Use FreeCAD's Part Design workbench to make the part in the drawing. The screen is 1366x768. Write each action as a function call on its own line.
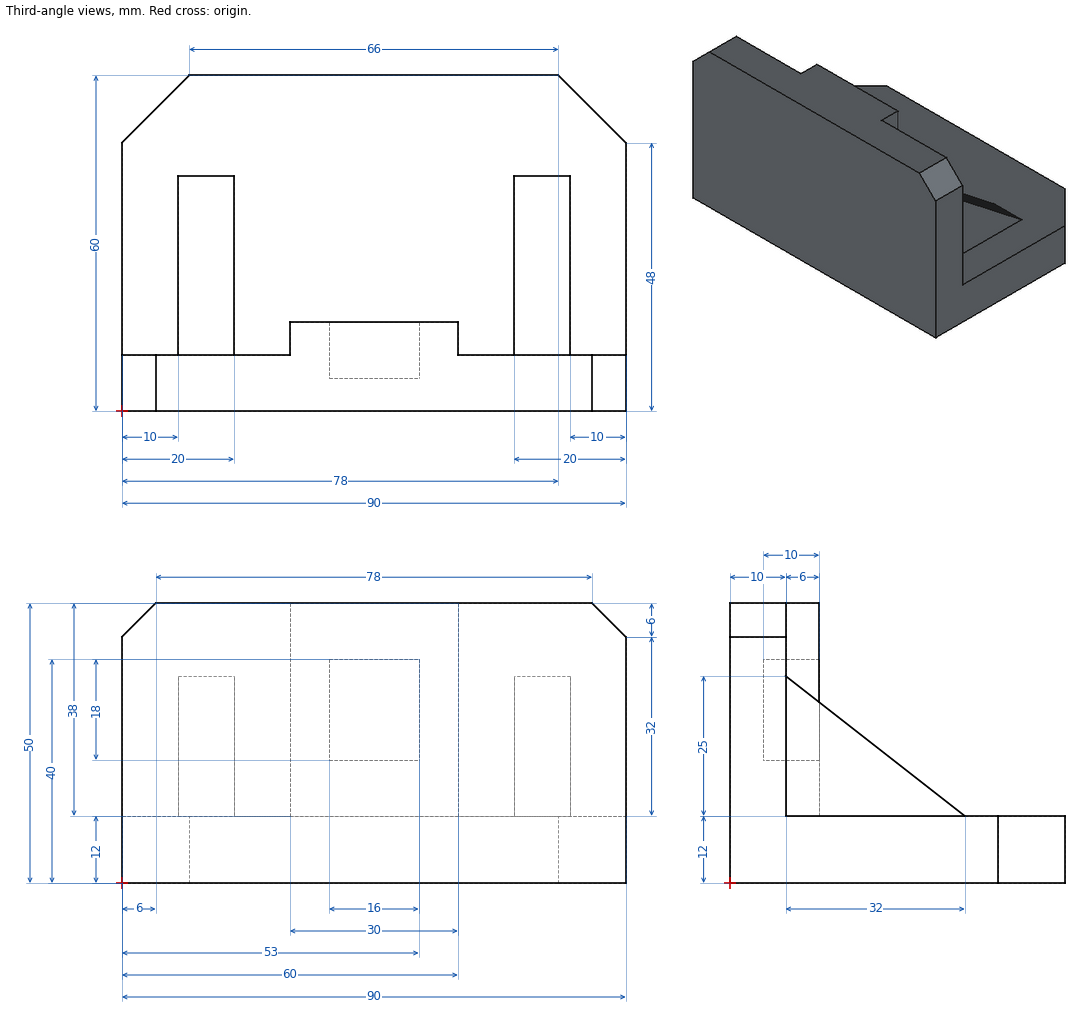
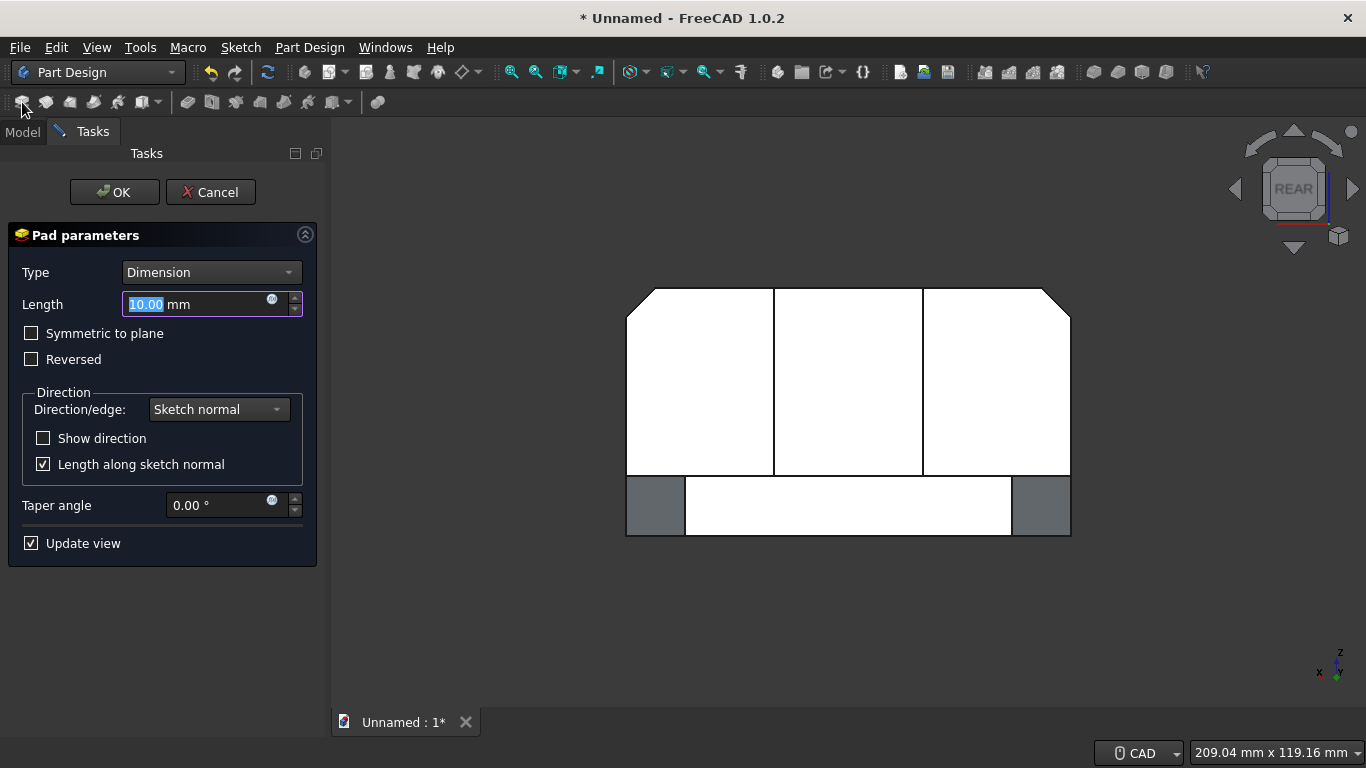
text(6)
key(Tab)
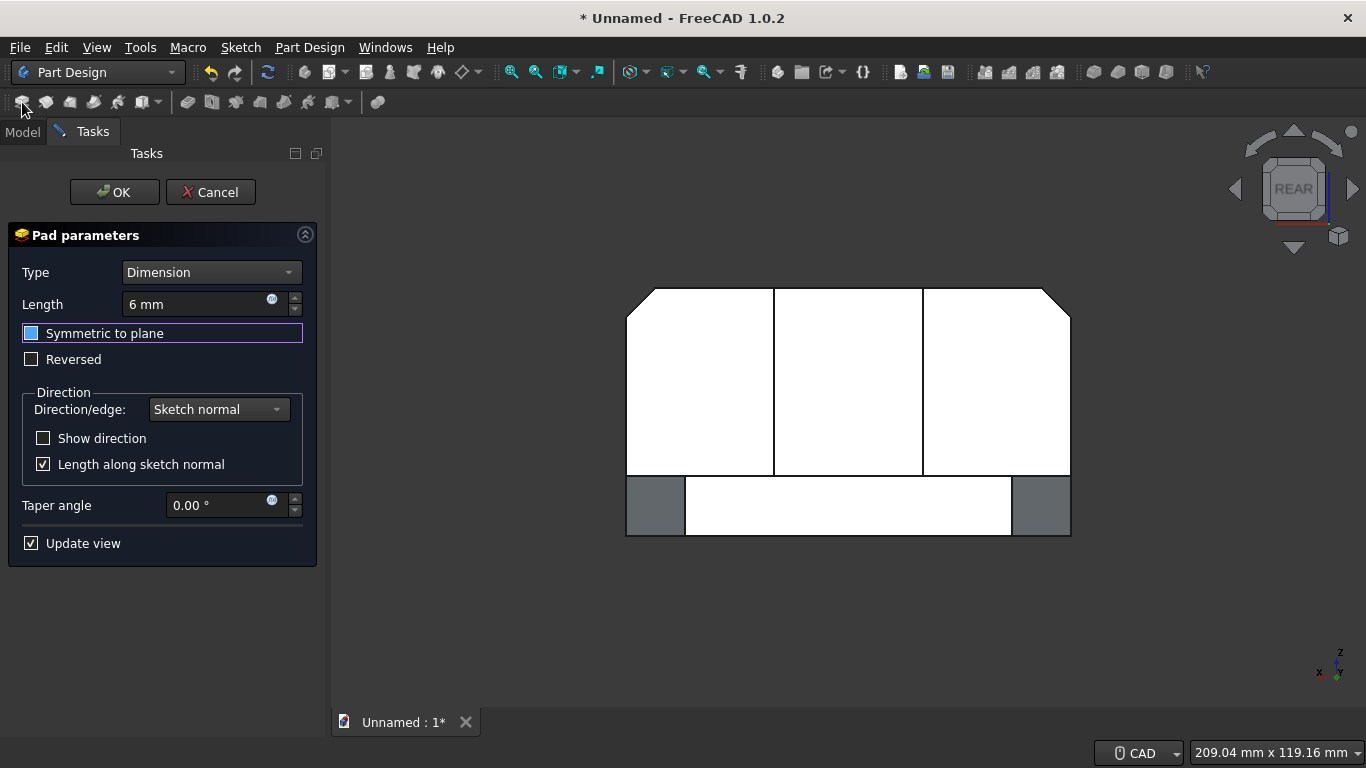
click(115, 192)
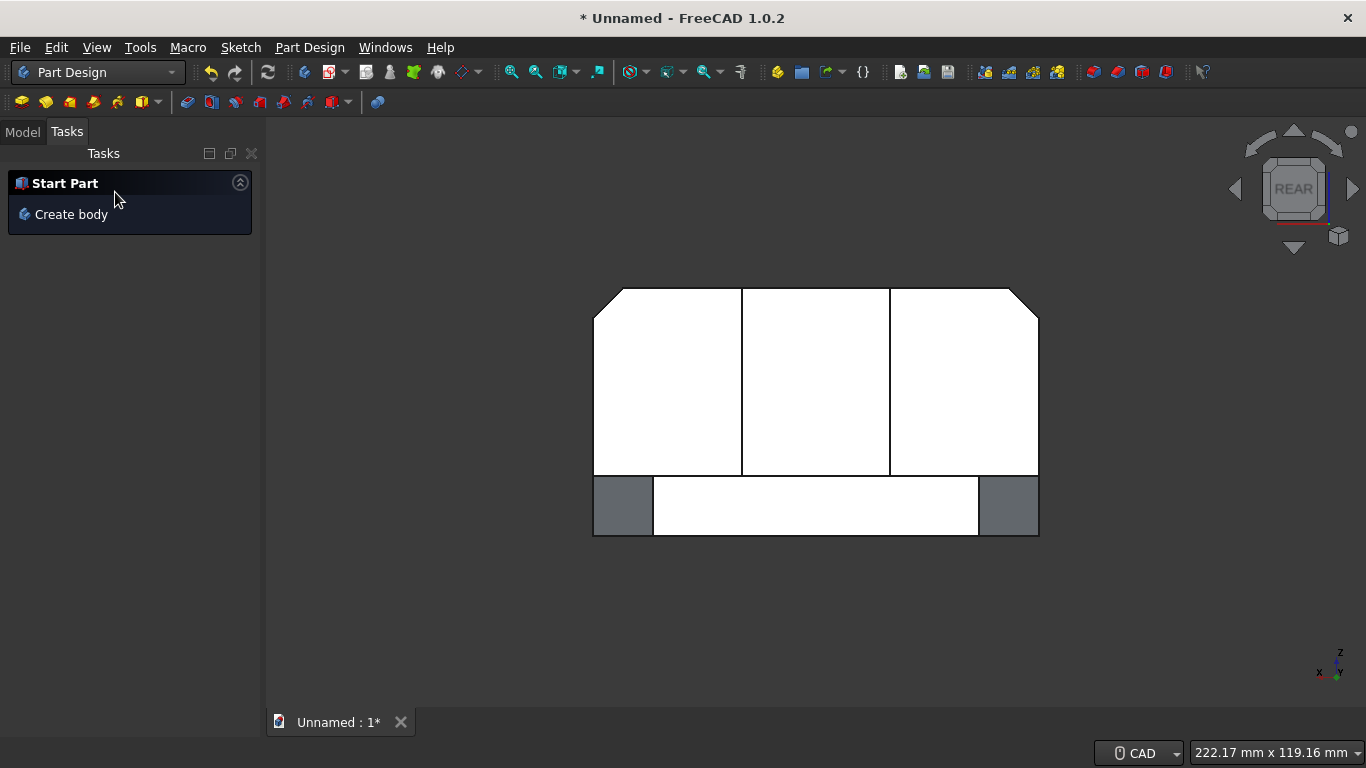
click(512, 72)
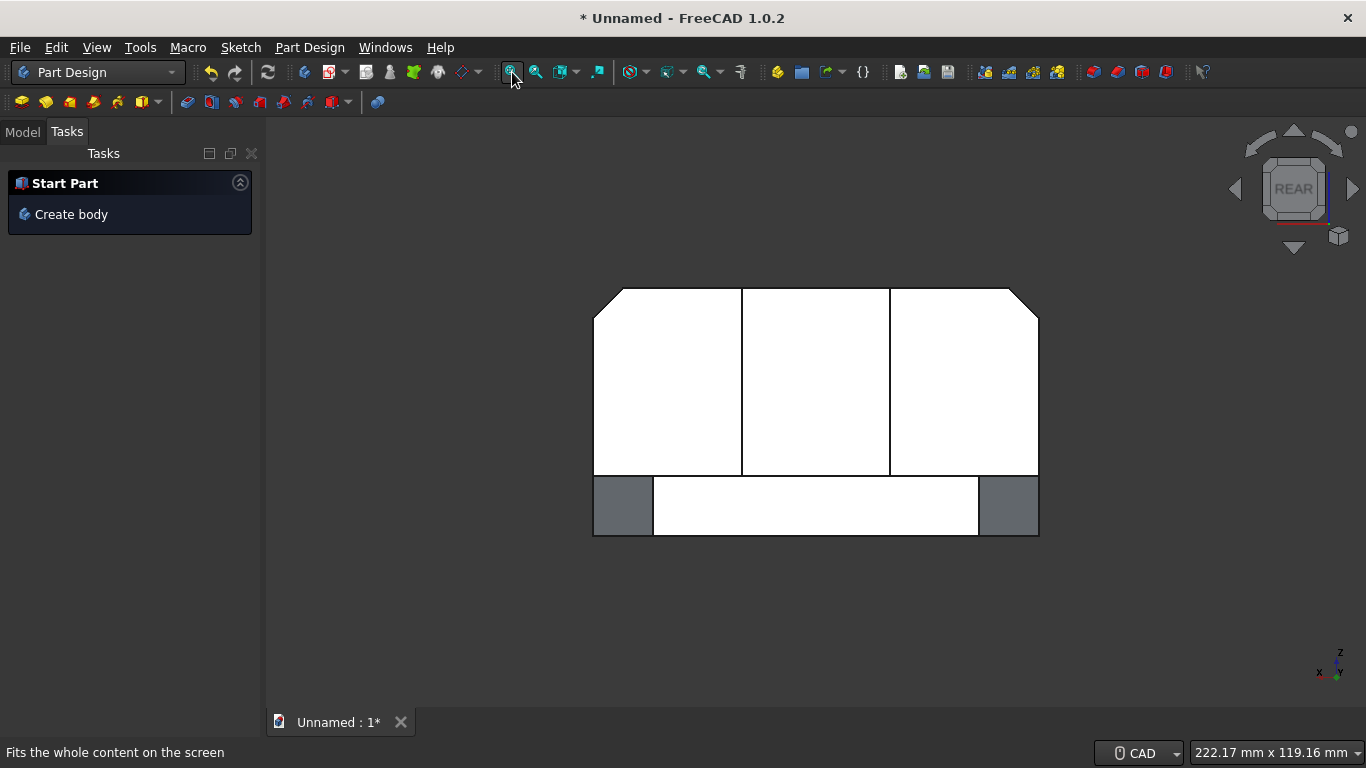
click(816, 381)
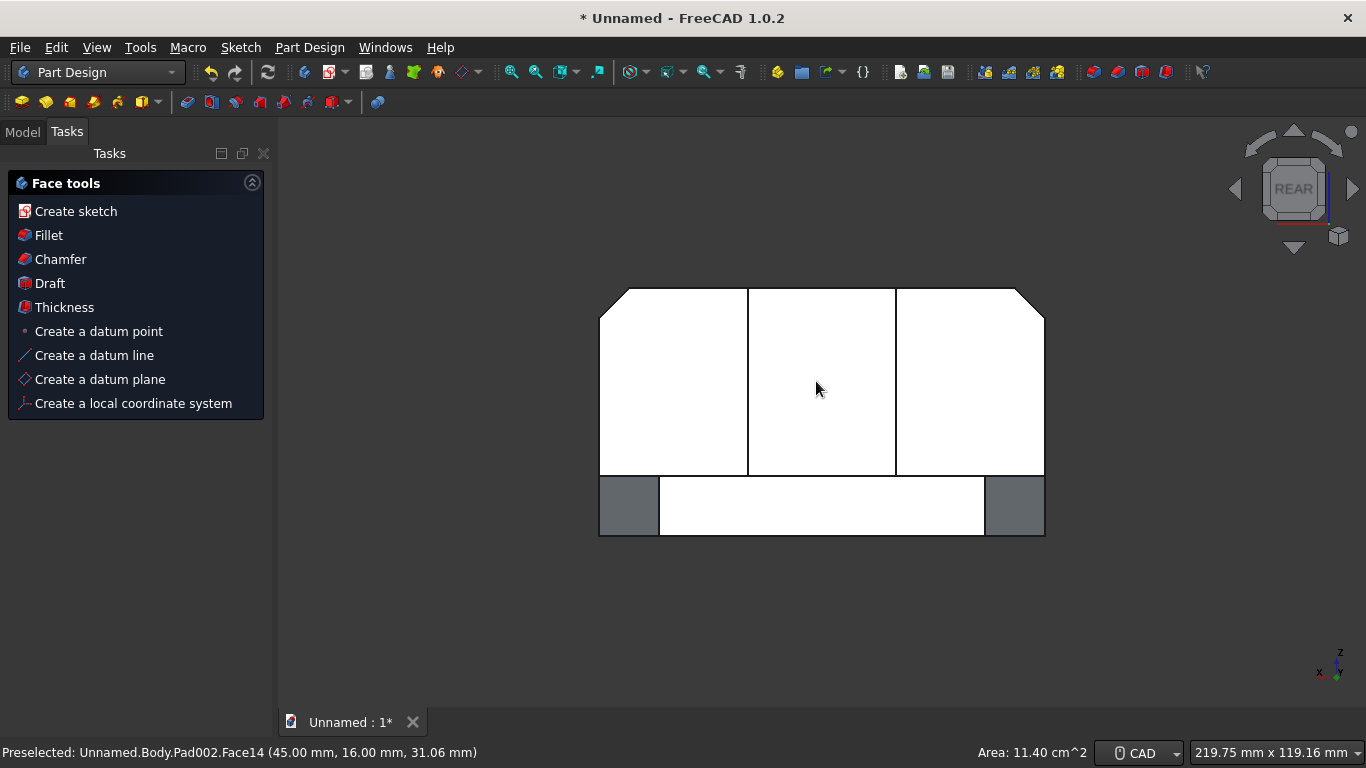
click(330, 72)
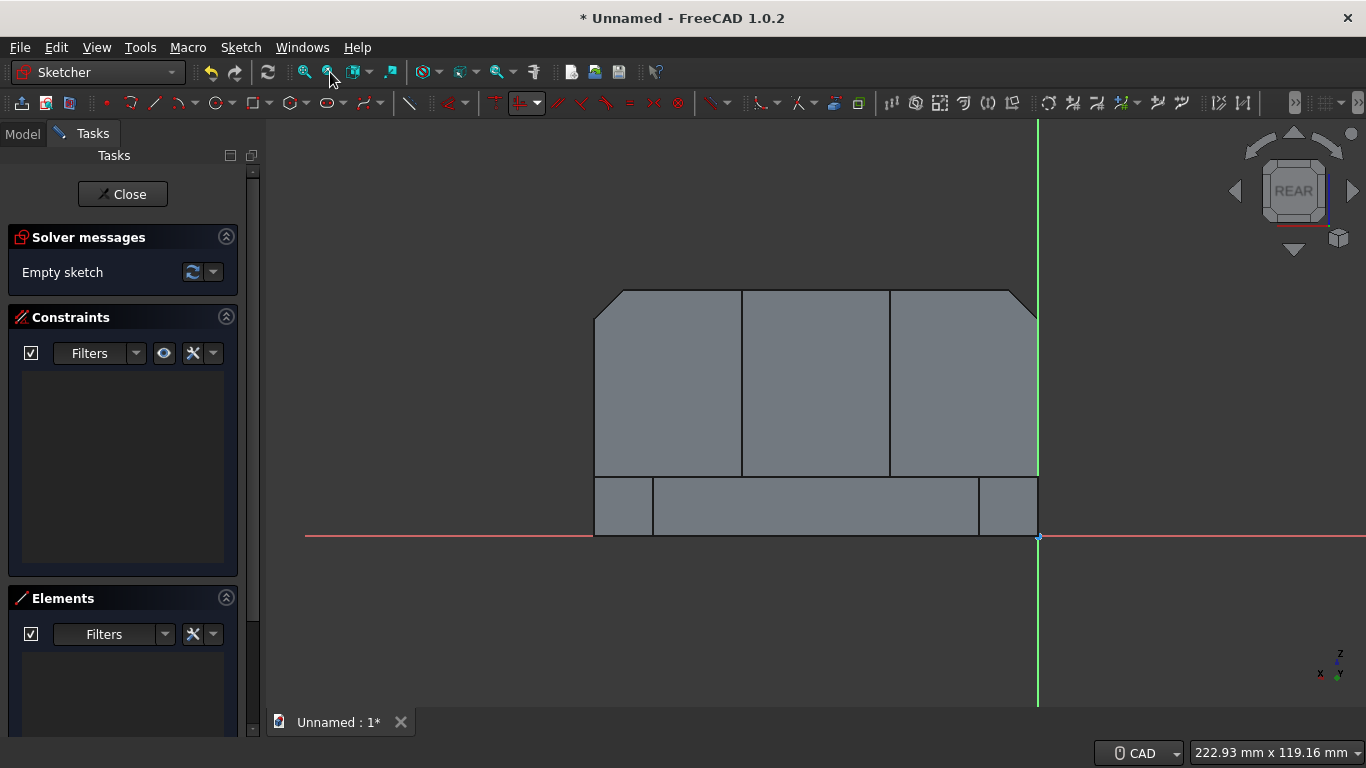
click(70, 104)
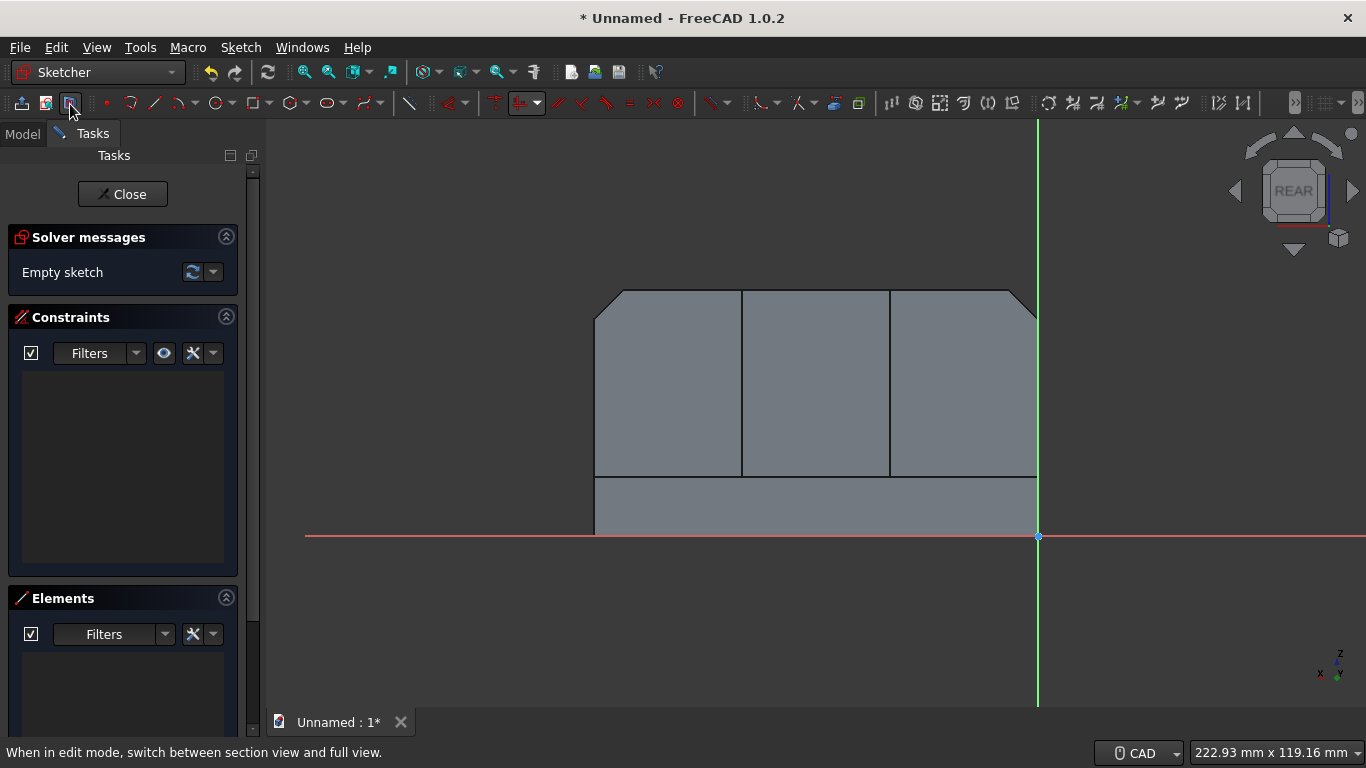
scroll(838, 374, up, 7)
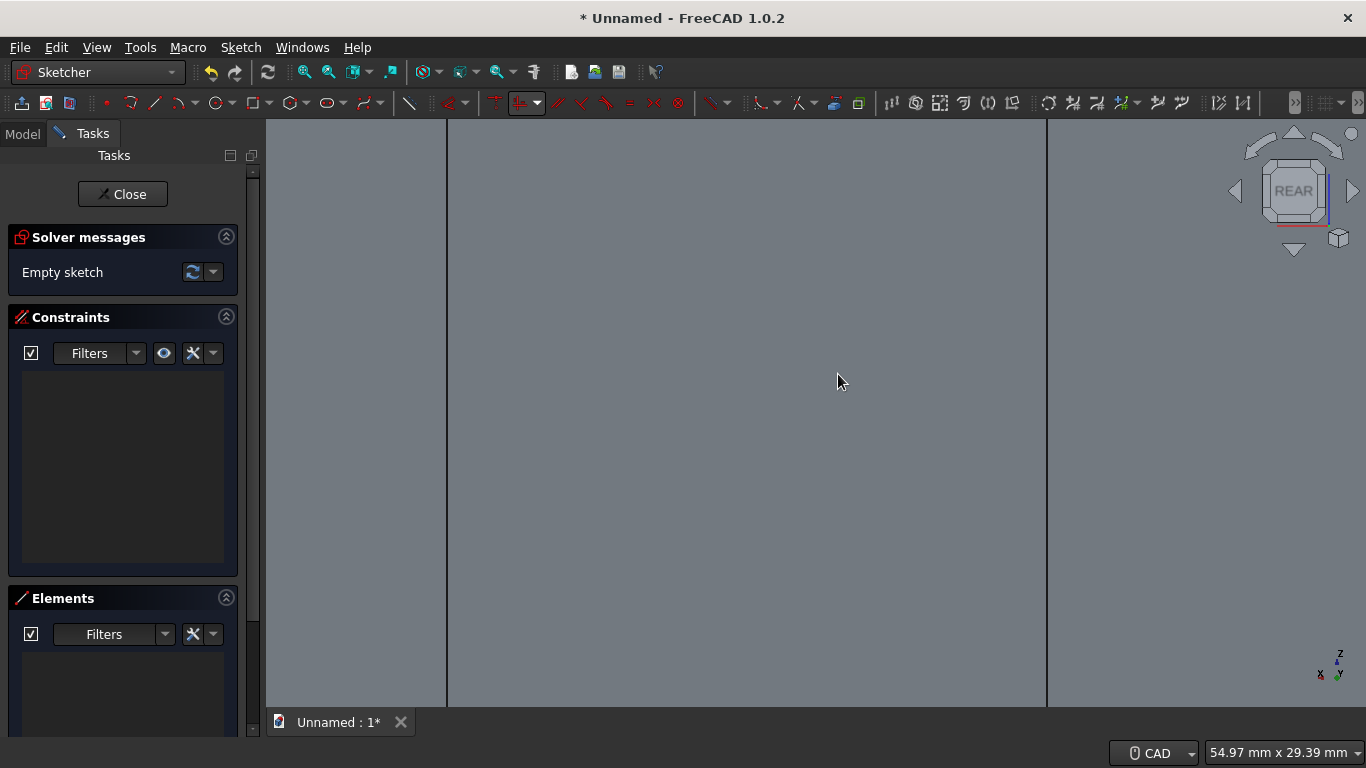
click(254, 104)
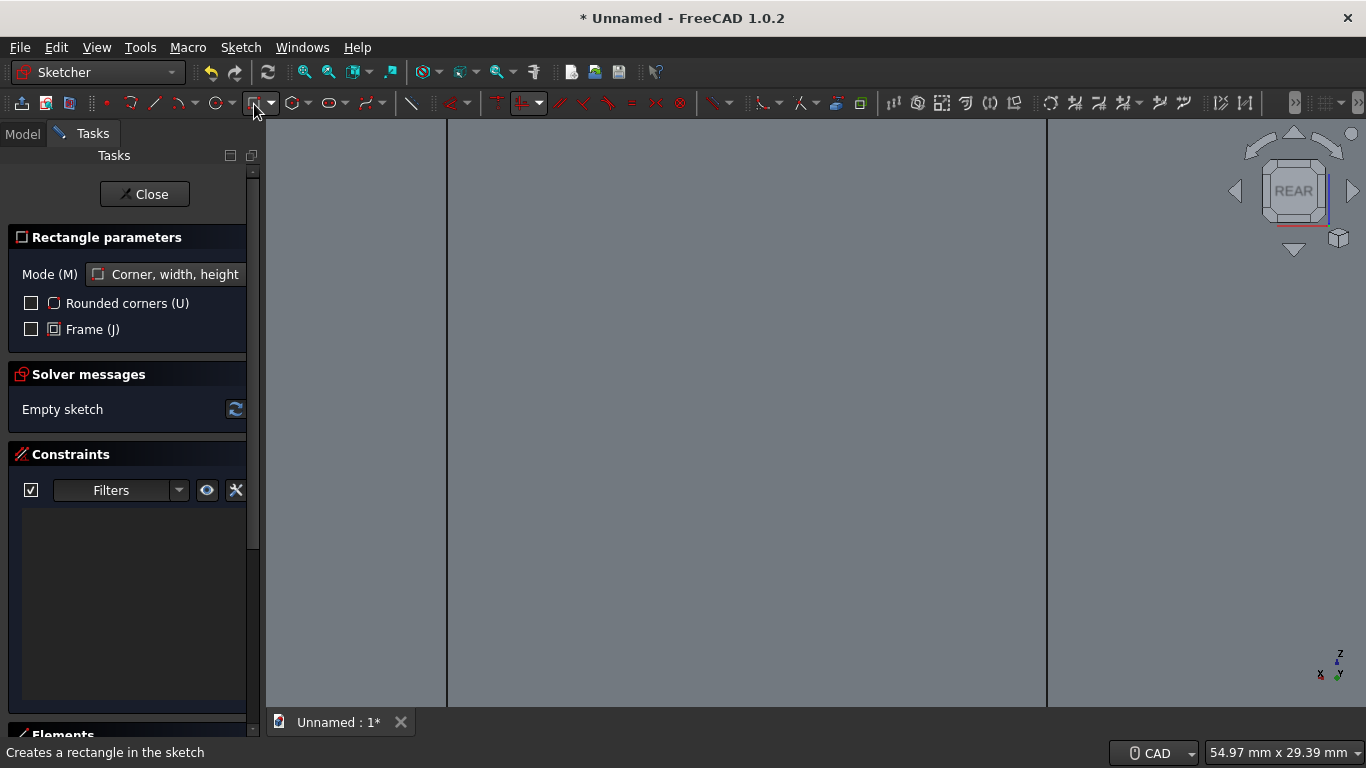
click(587, 231)
move(907, 591)